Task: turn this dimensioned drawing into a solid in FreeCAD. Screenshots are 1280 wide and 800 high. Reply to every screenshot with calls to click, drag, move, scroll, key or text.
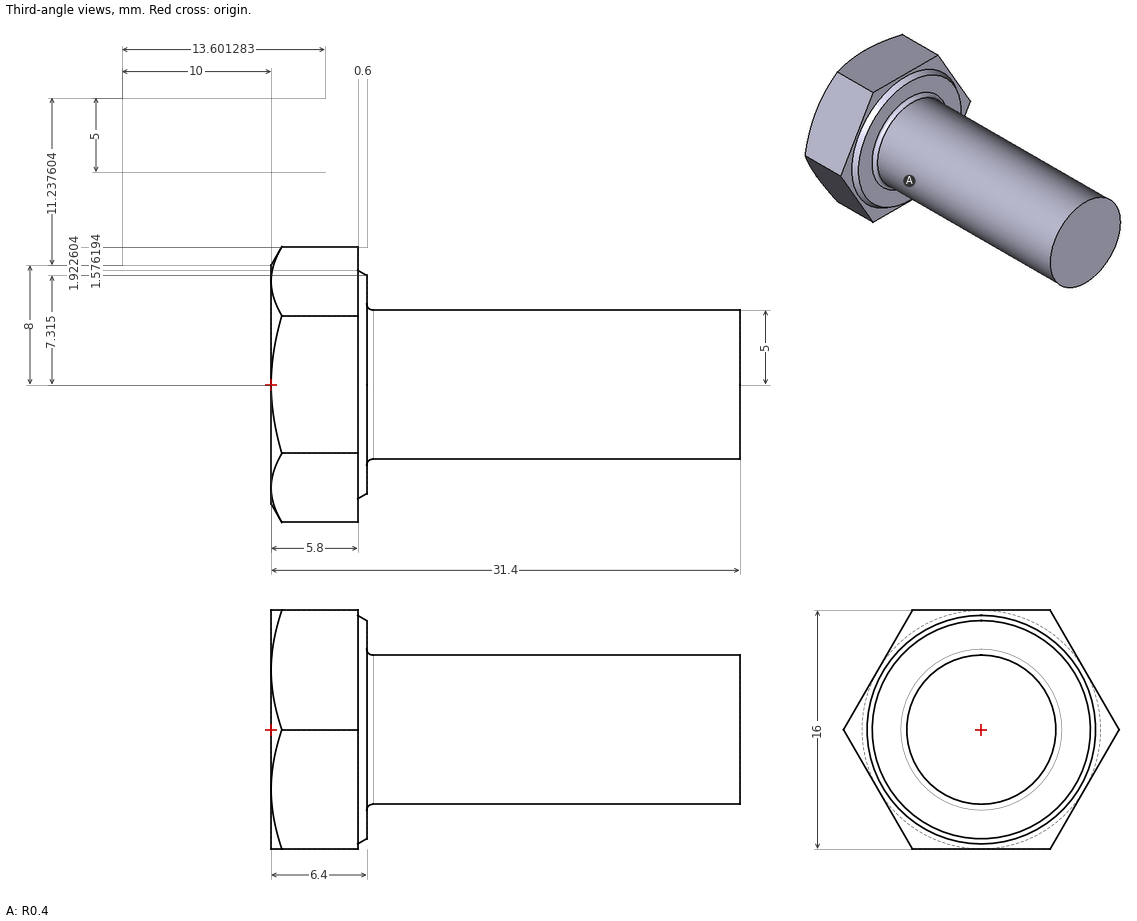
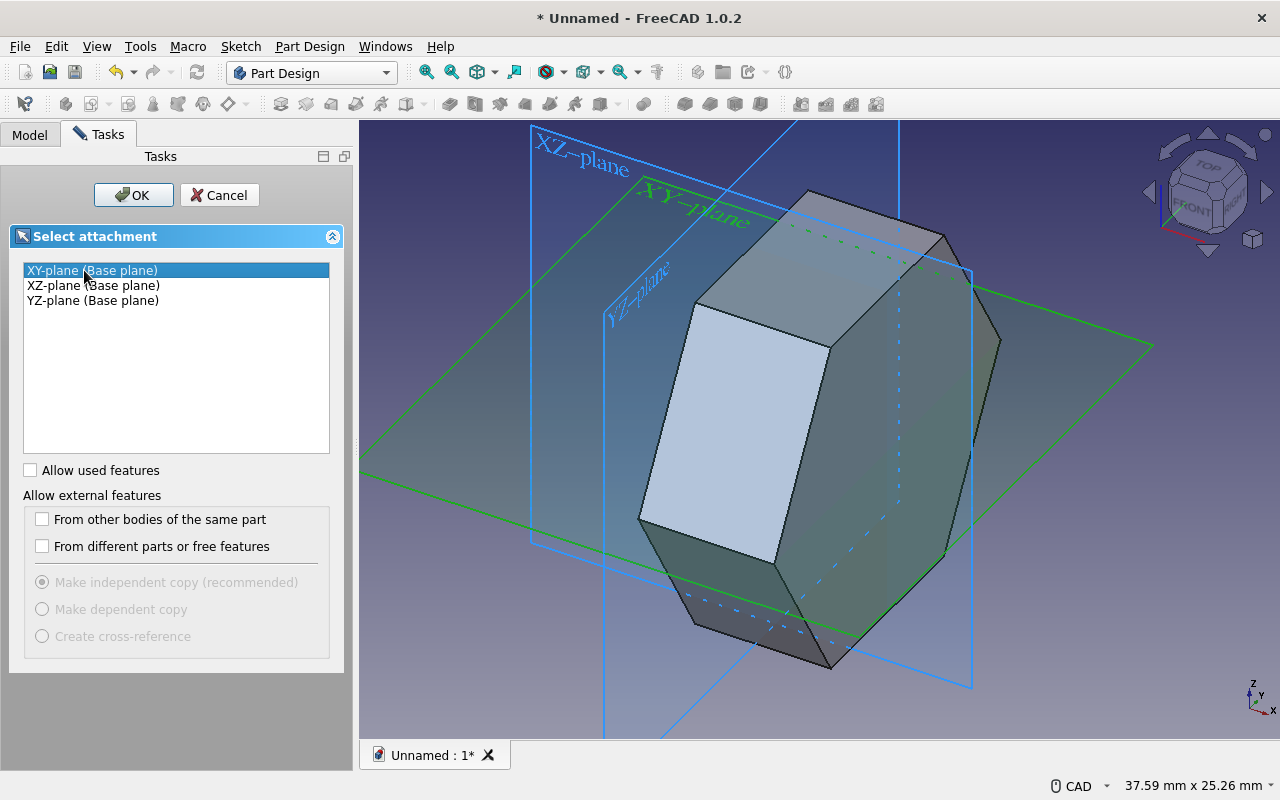
click(134, 195)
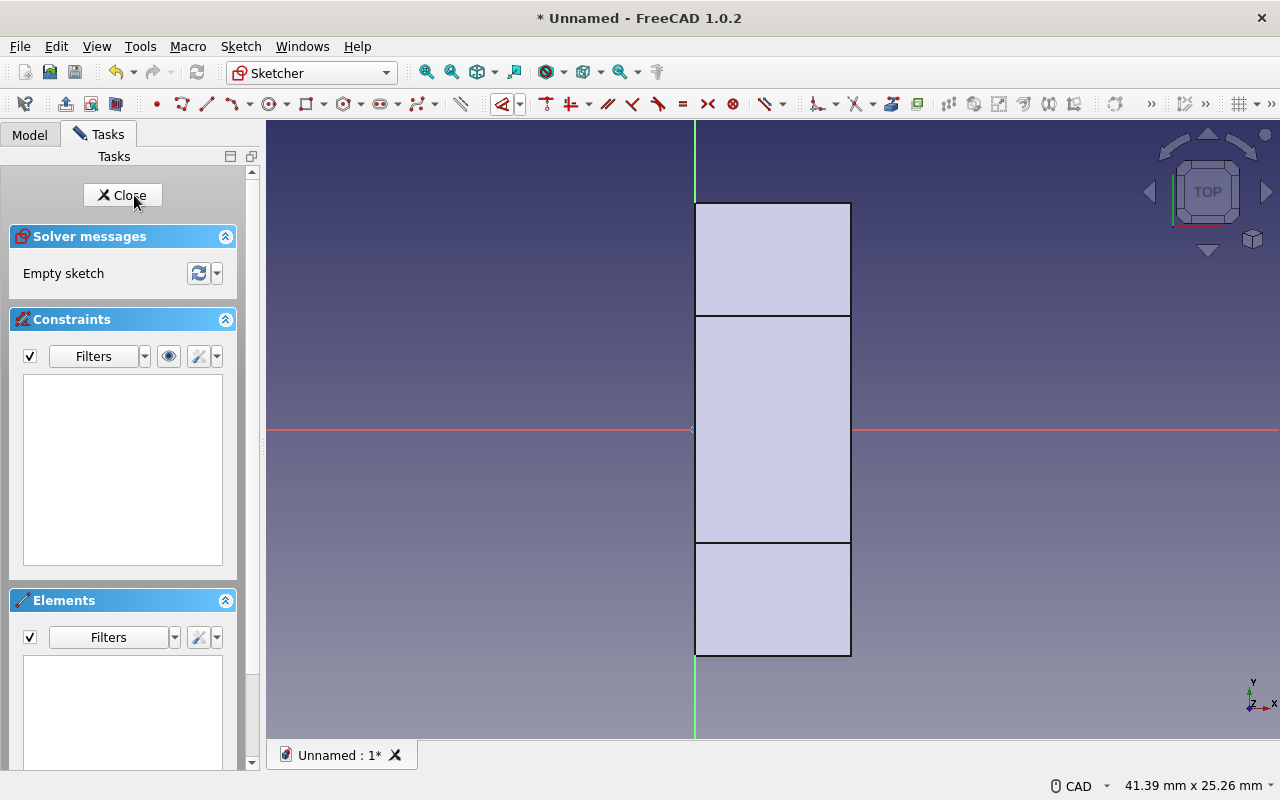
key(q)
key(s)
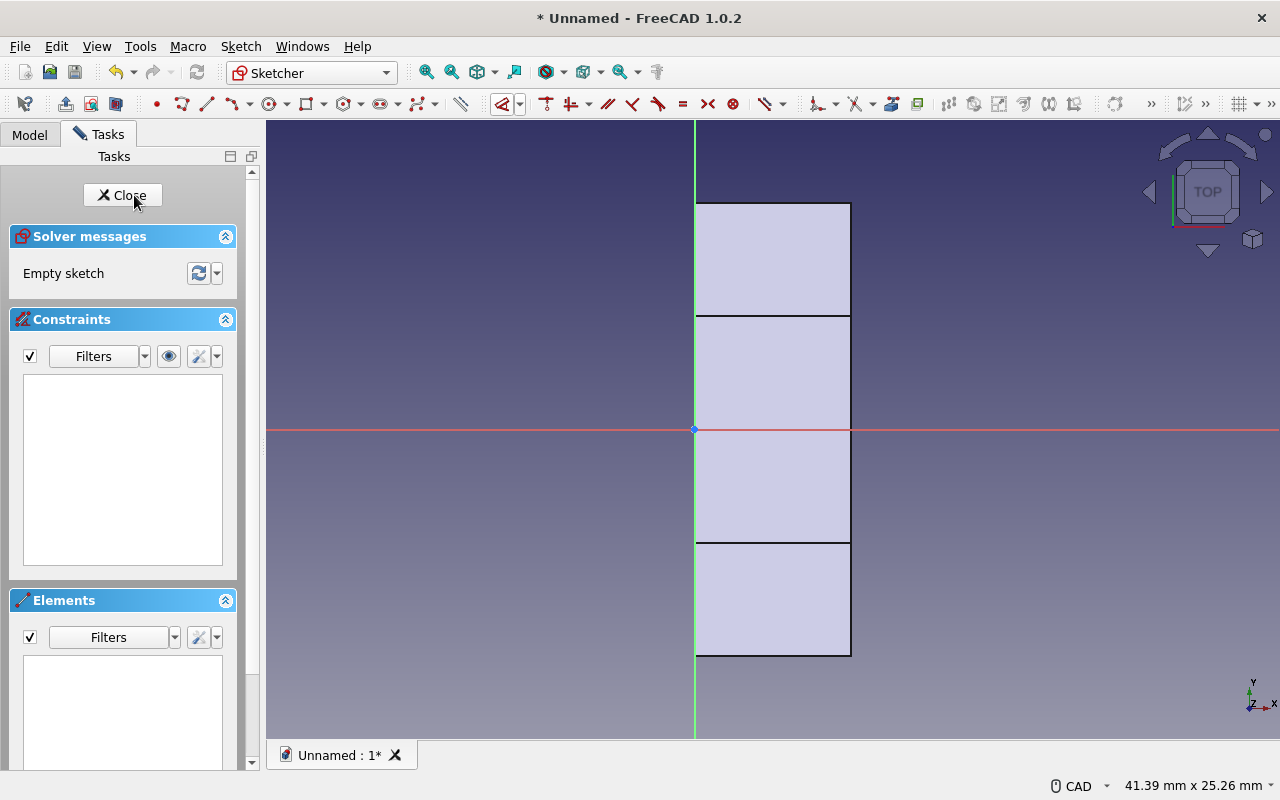
scroll(294, 554, down, 2)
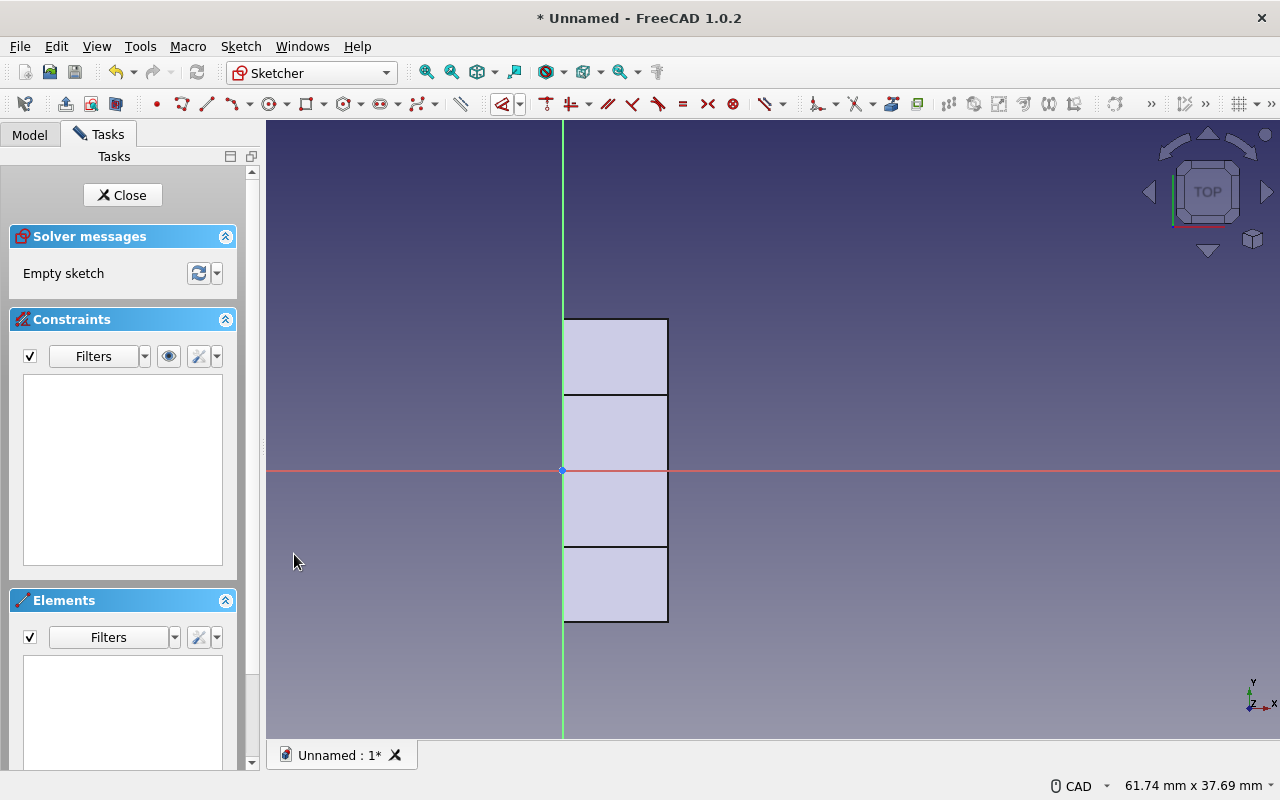
click(306, 104)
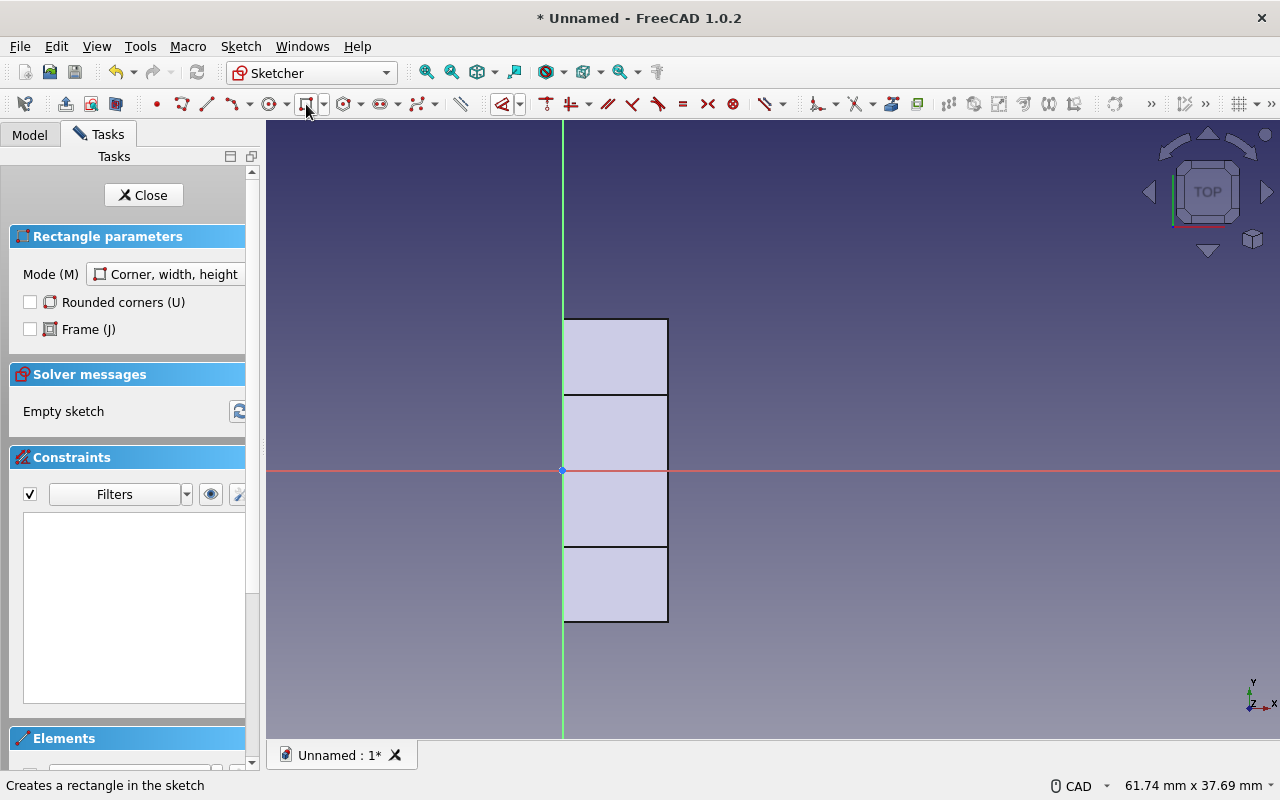
click(563, 471)
move(1078, 389)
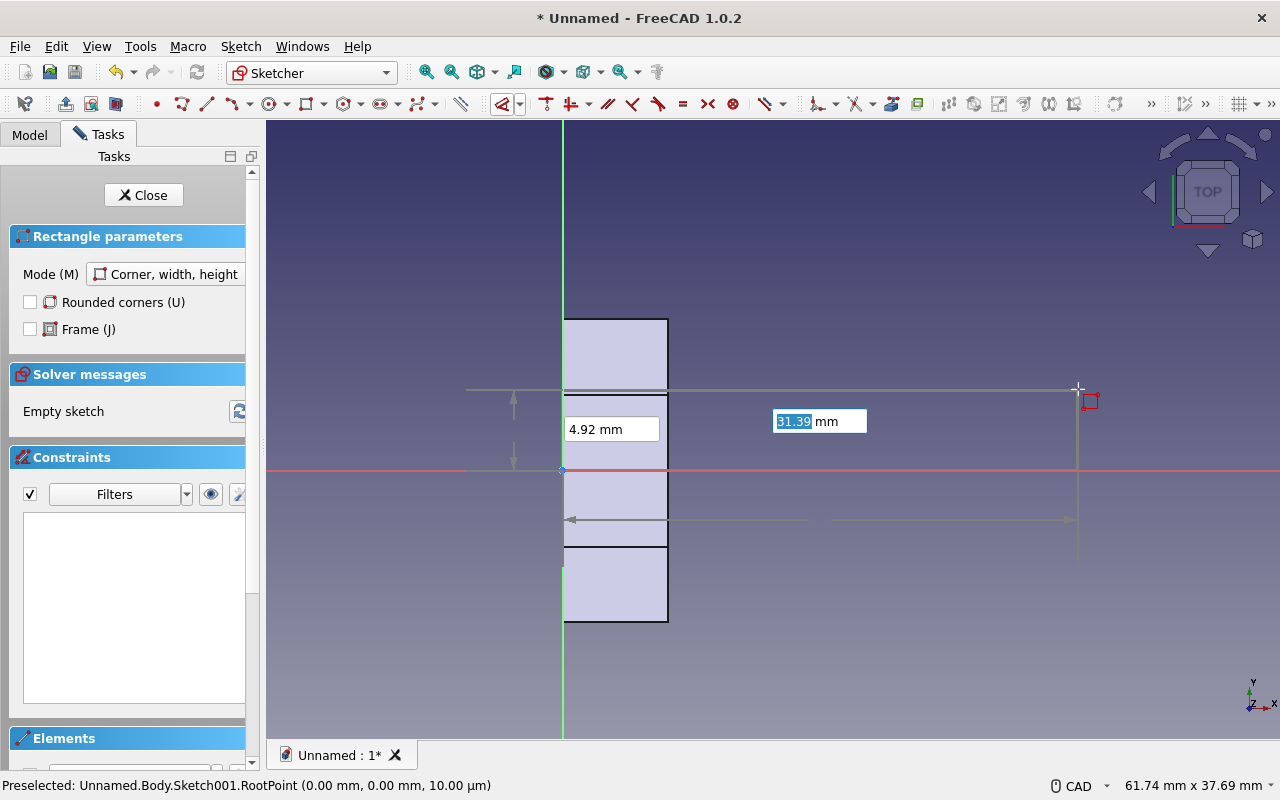
text(31.4)
key(Tab)
text(5)
key(Return)
key(Escape)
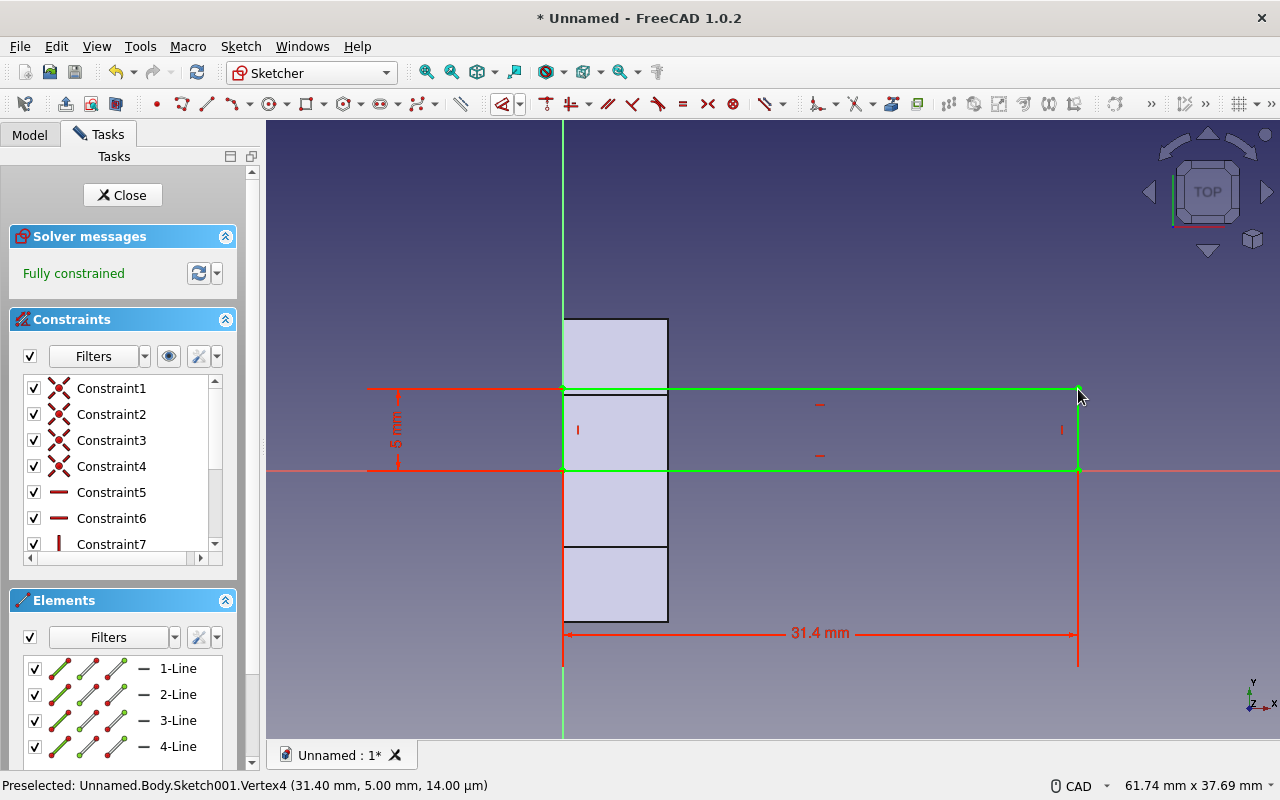
click(123, 195)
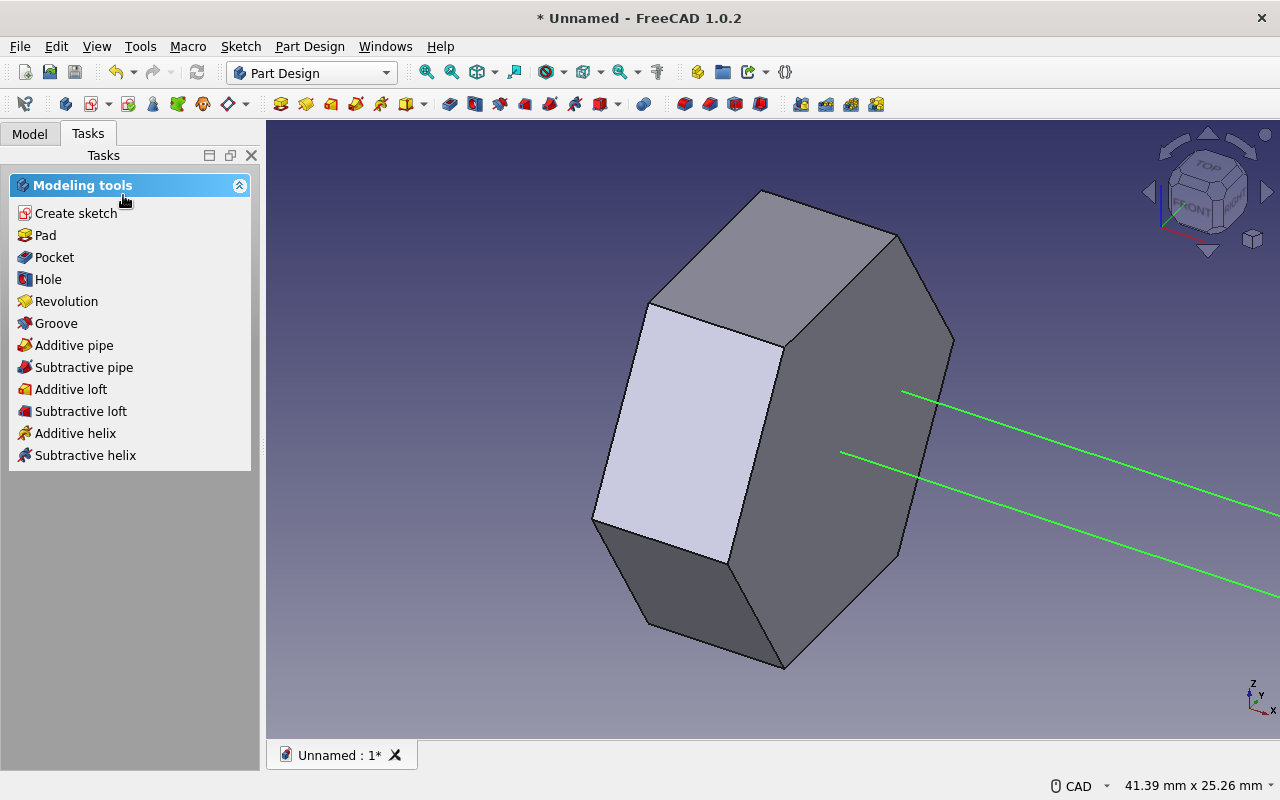
click(306, 104)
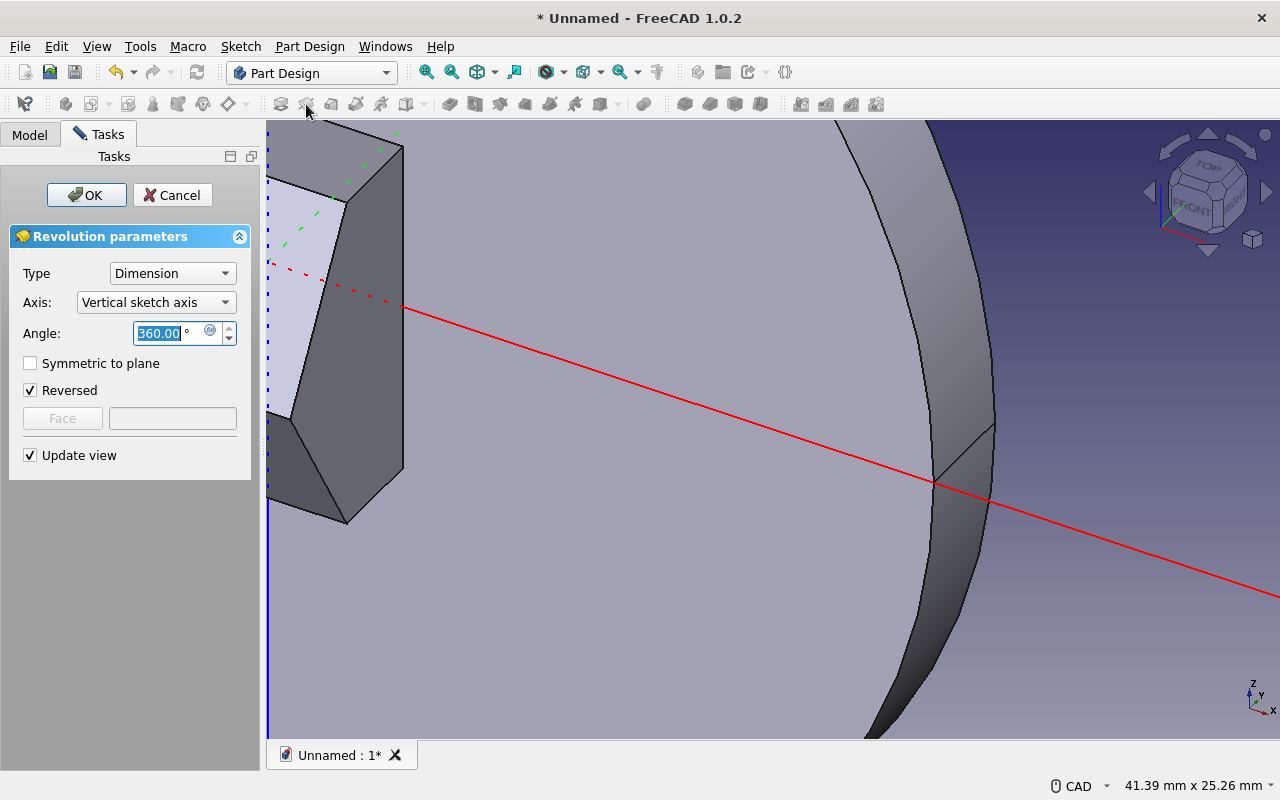
click(157, 302)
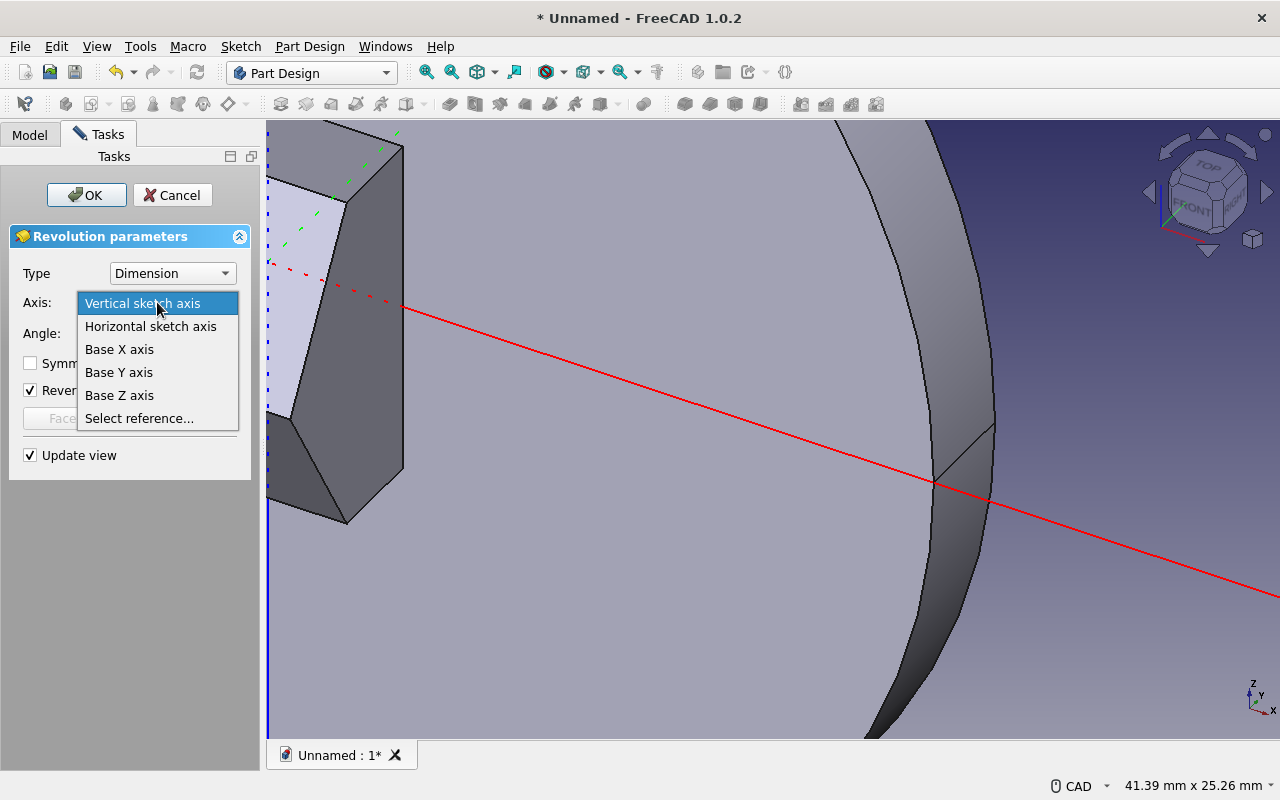
click(156, 326)